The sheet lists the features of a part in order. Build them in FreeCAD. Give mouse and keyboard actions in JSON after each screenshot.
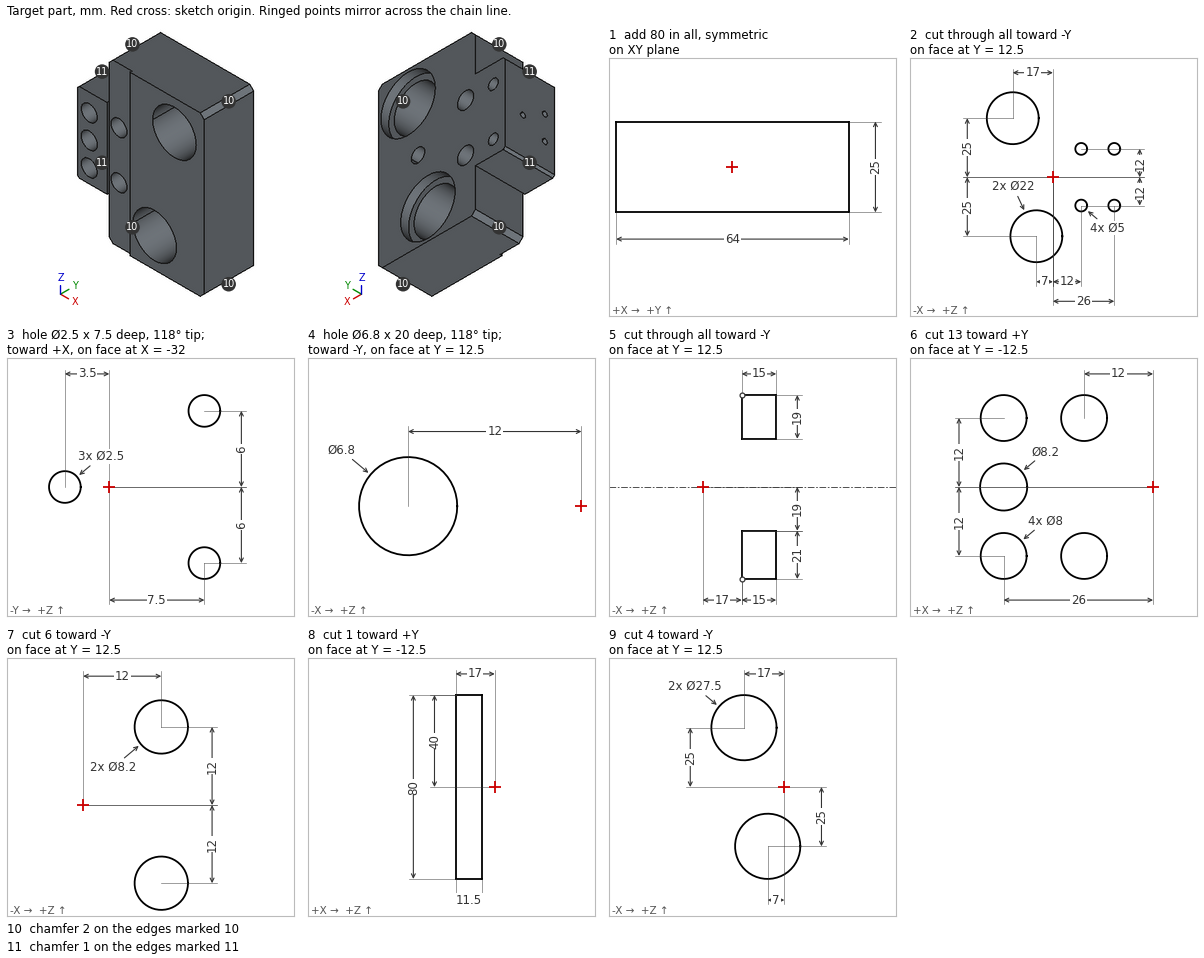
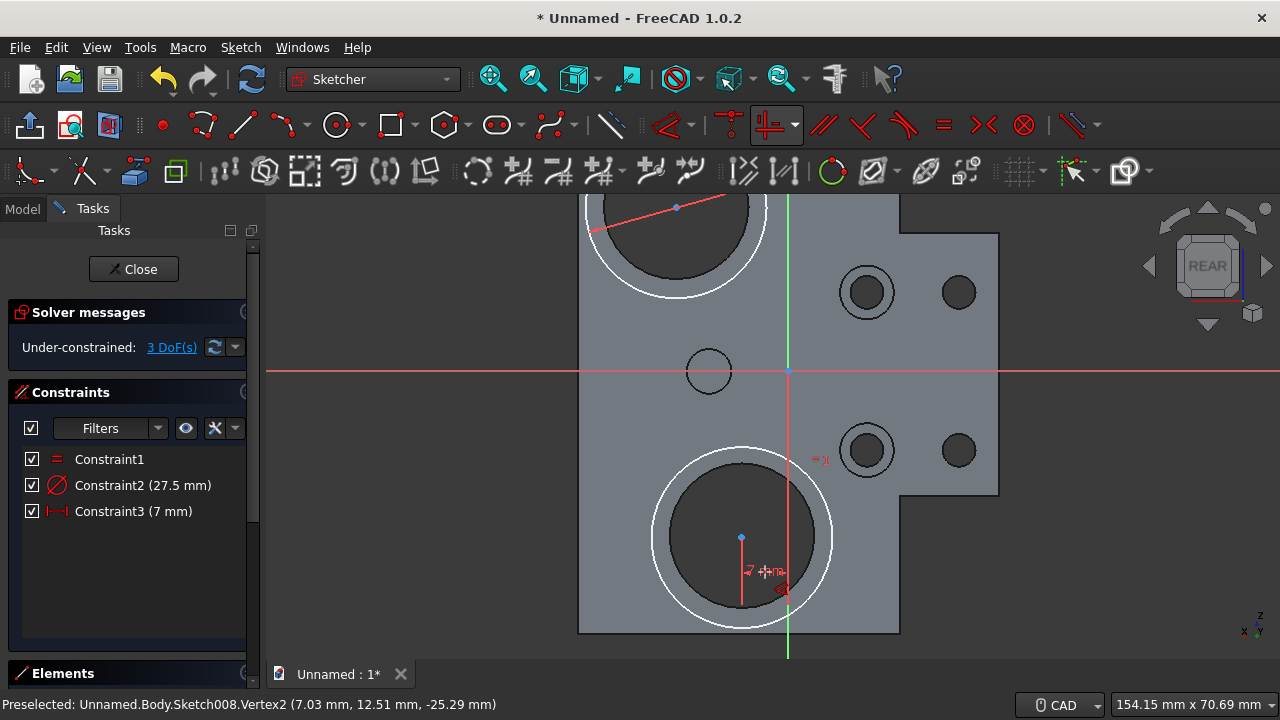
{"action": "scroll", "coordinate": [699, 494], "scroll_direction": "down", "scroll_amount": 3}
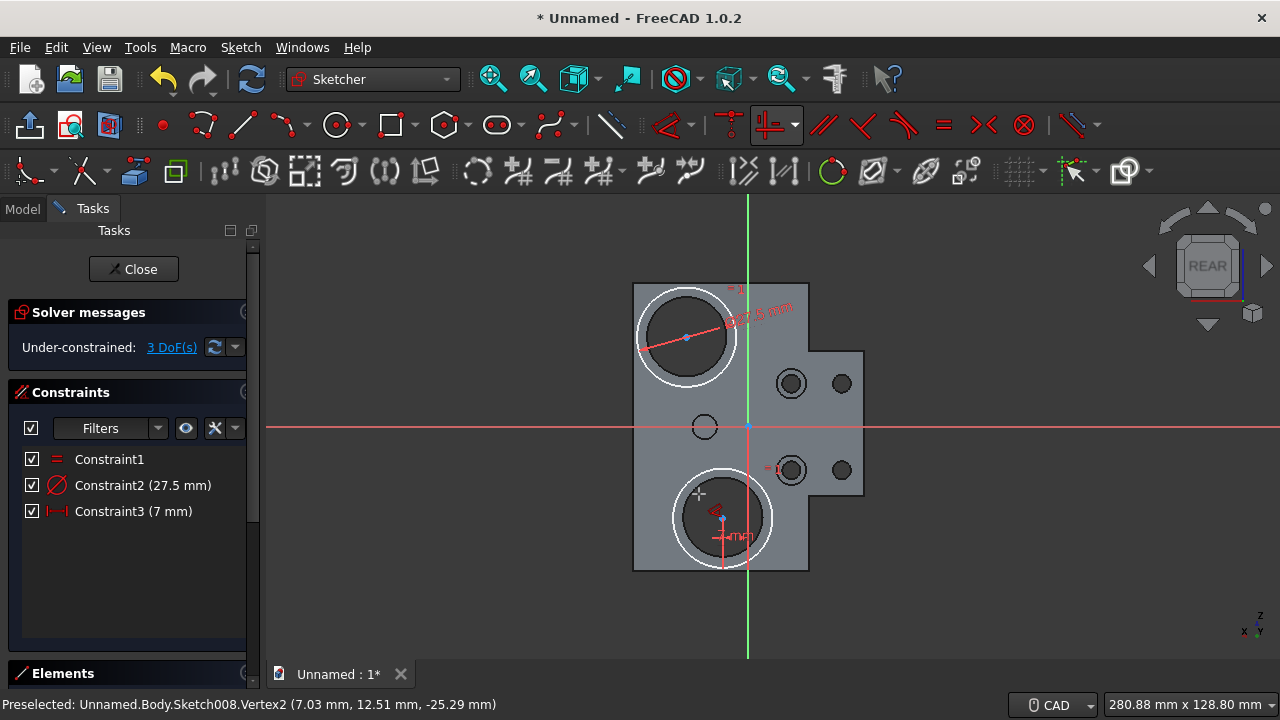
{"action": "left_click", "coordinate": [687, 337]}
{"action": "left_click", "coordinate": [696, 461]}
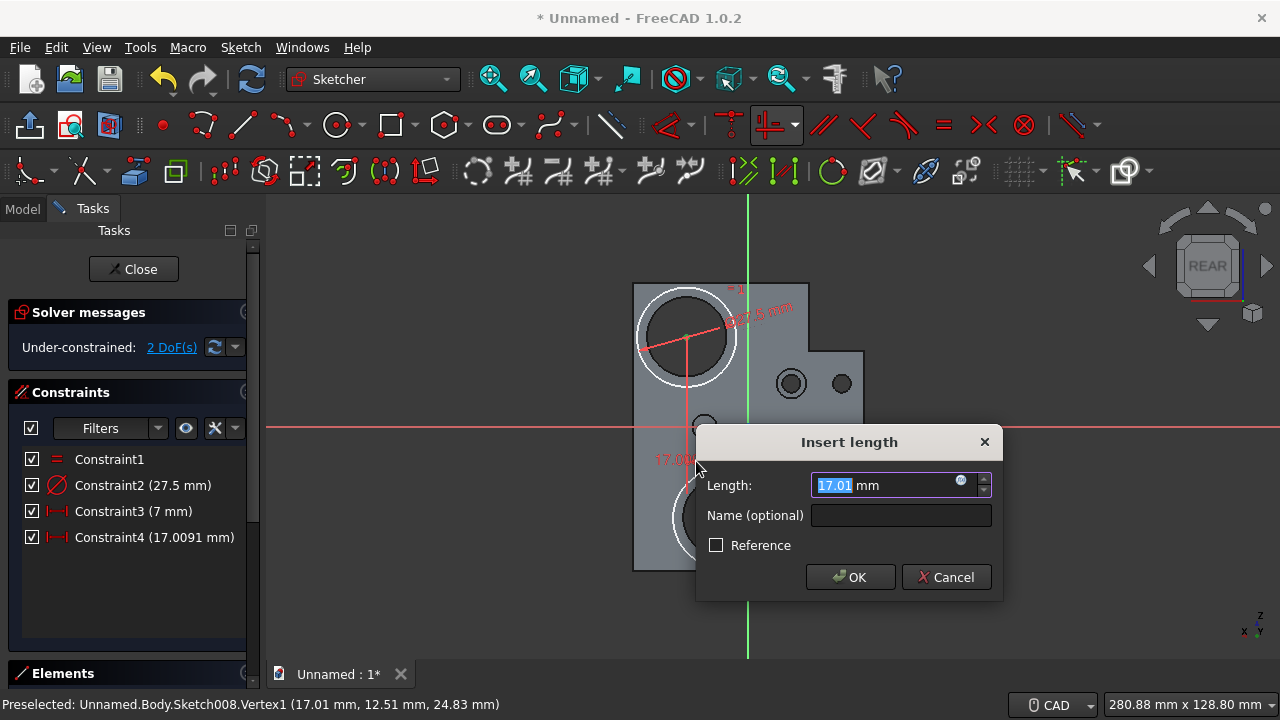
{"action": "type", "text": "17"}
{"action": "key", "text": "Return"}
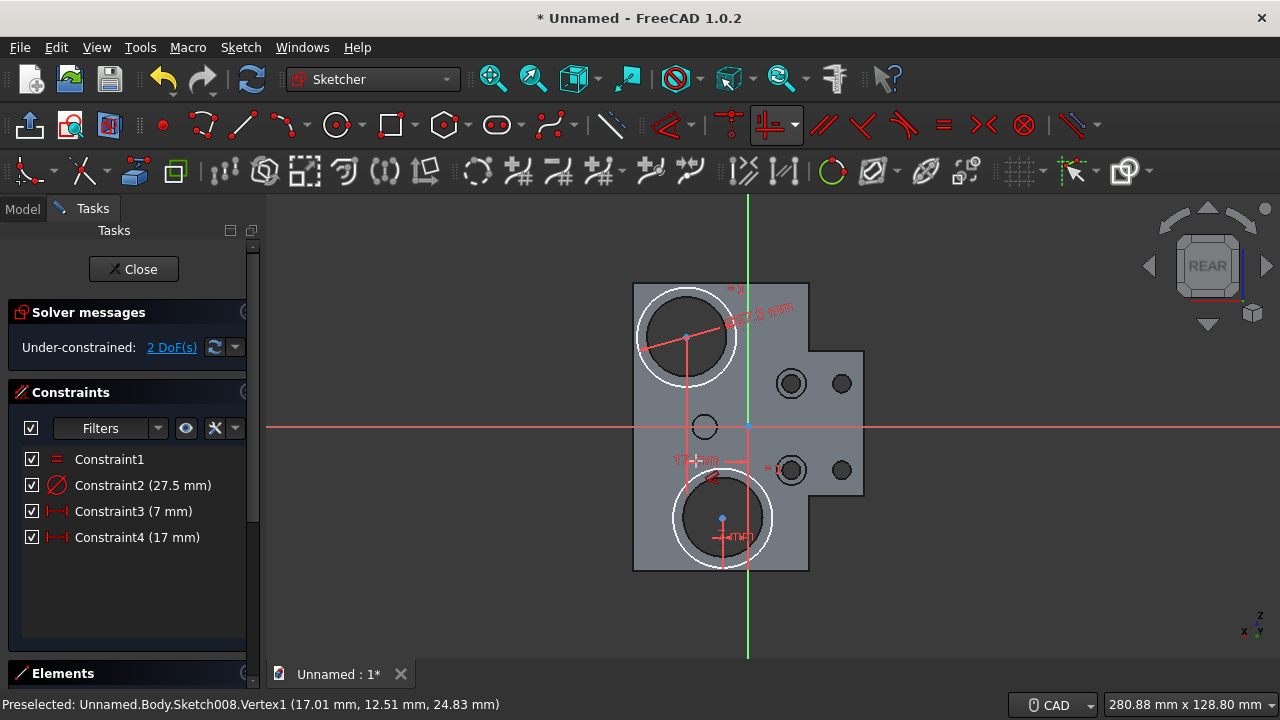
{"action": "left_click", "coordinate": [687, 337]}
{"action": "left_click", "coordinate": [782, 382]}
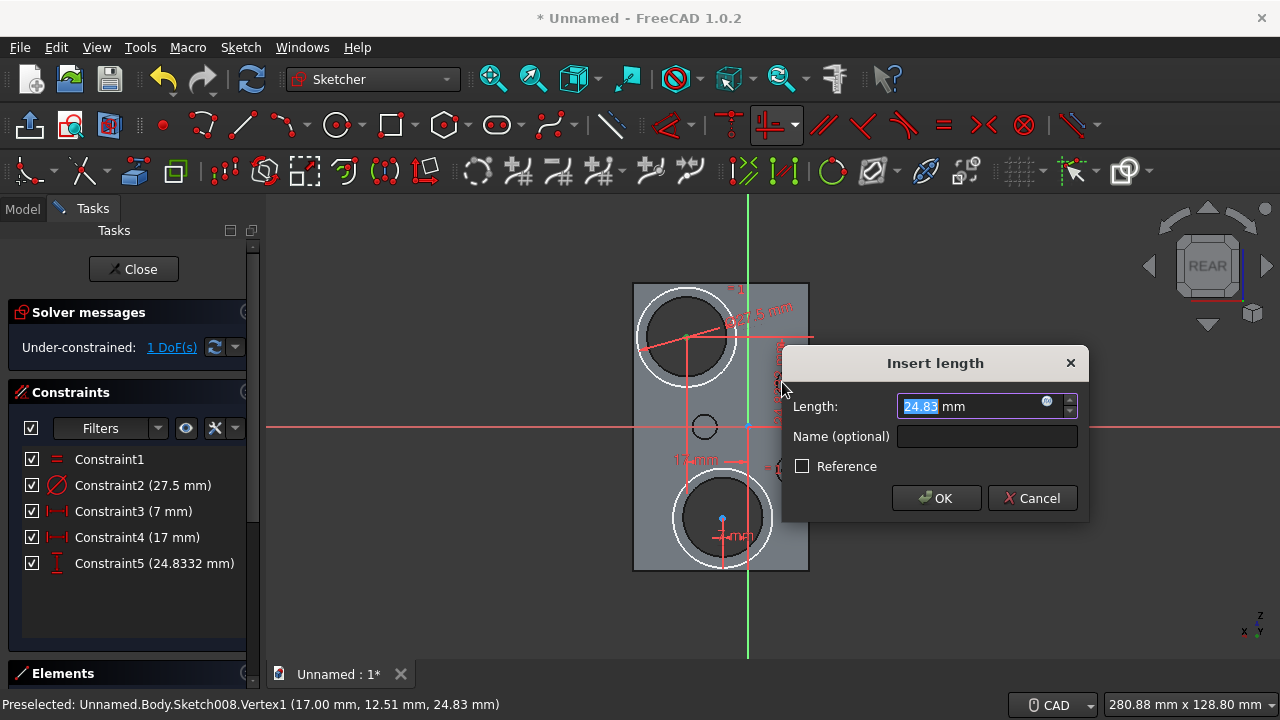
{"action": "type", "text": "25"}
{"action": "key", "text": "Return"}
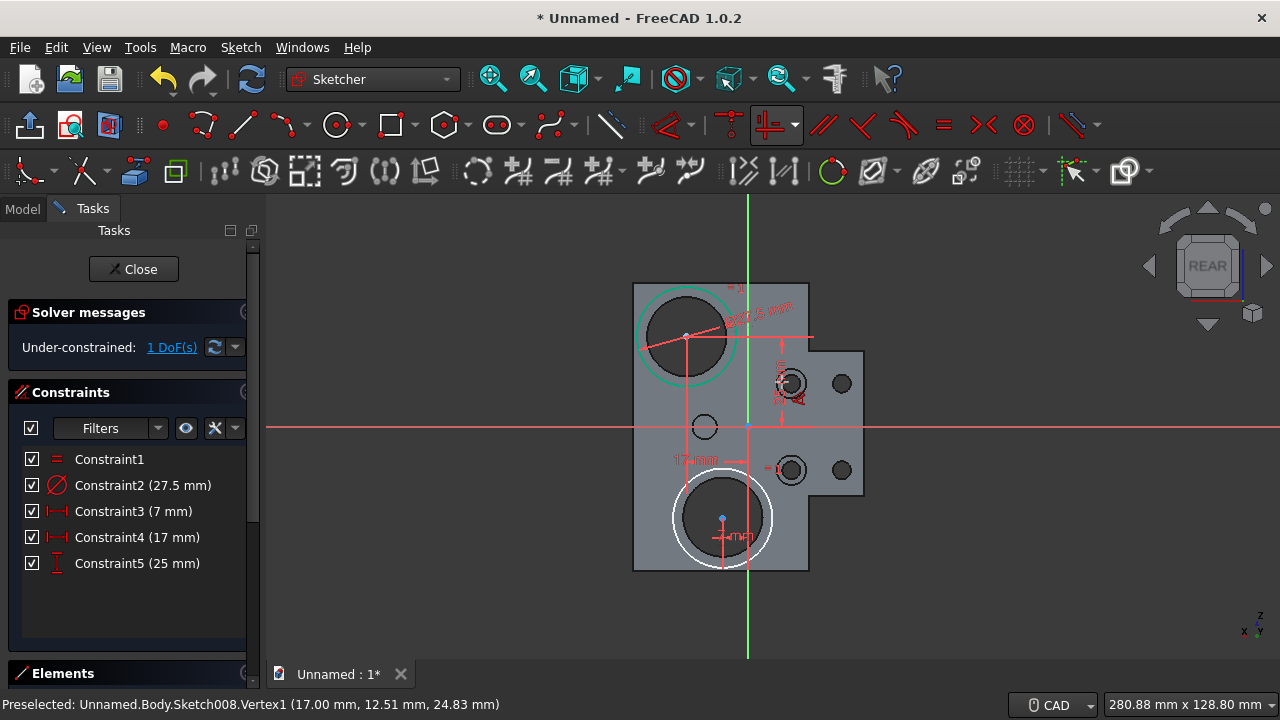
{"action": "left_click", "coordinate": [723, 518]}
{"action": "left_click", "coordinate": [782, 473]}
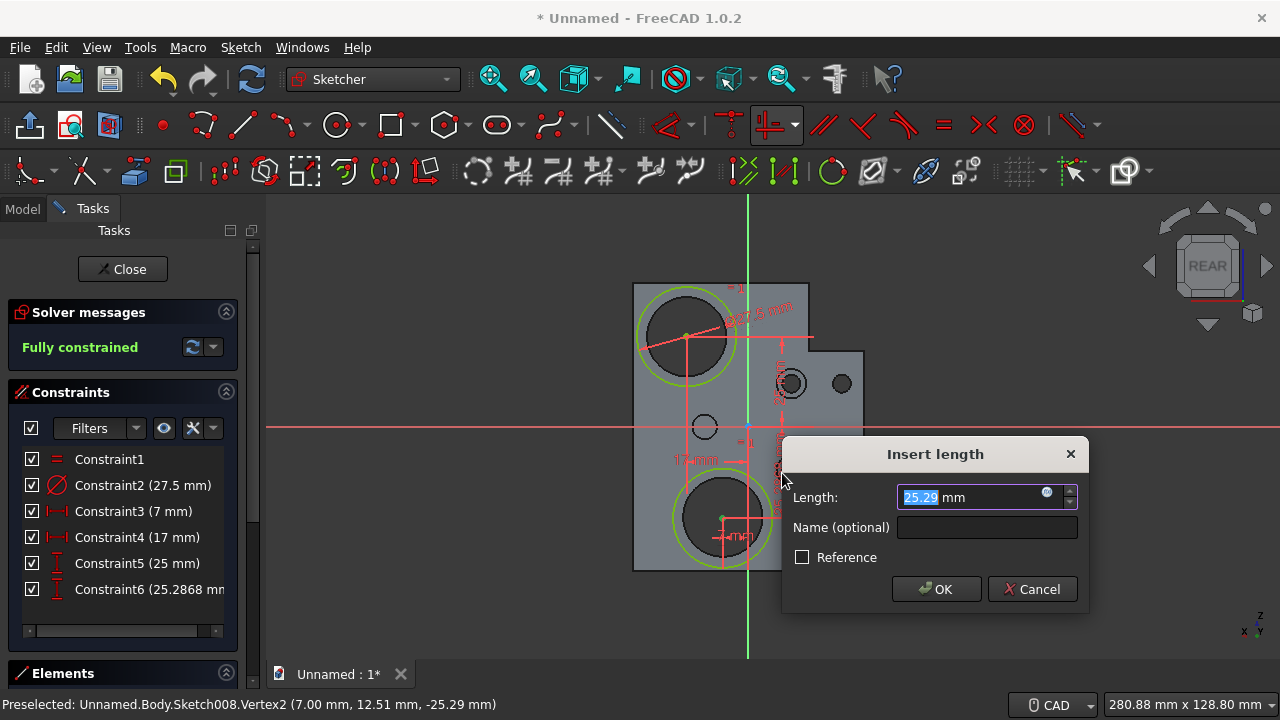
{"action": "type", "text": "25"}
{"action": "key", "text": "Return"}
{"action": "key", "text": "Escape"}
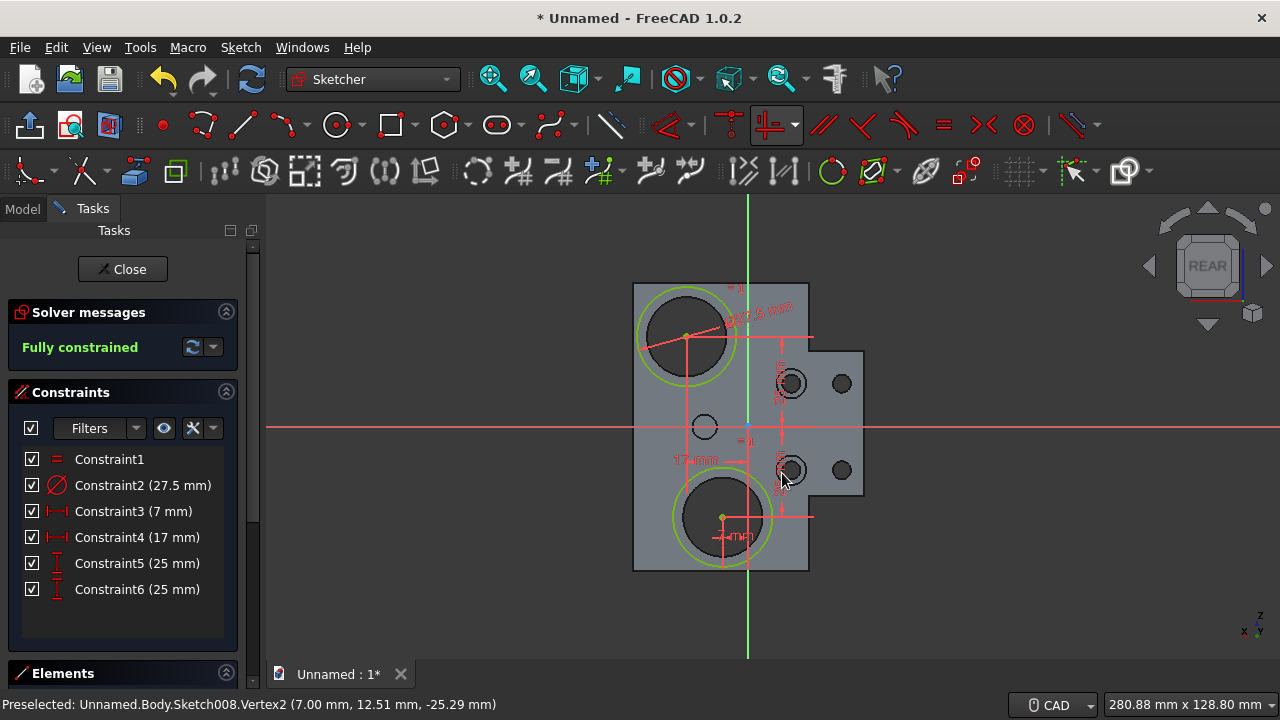
{"action": "left_click", "coordinate": [123, 269]}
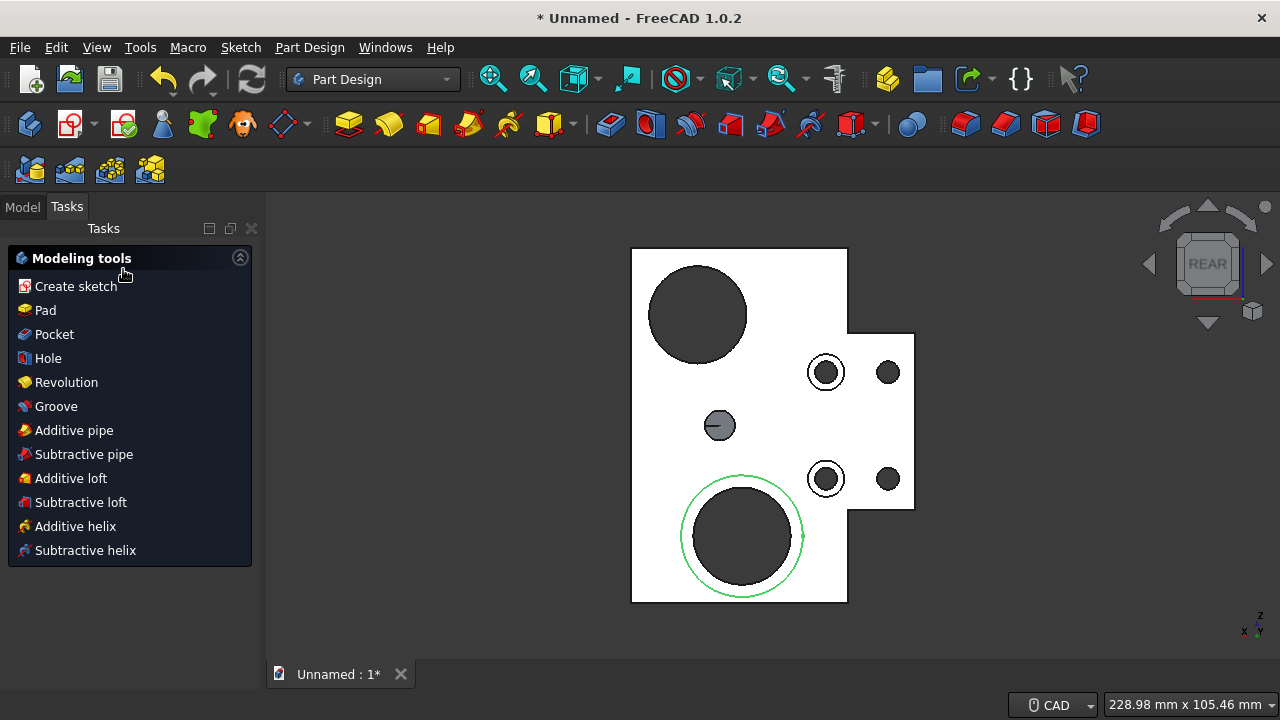
{"action": "left_click", "coordinate": [612, 124]}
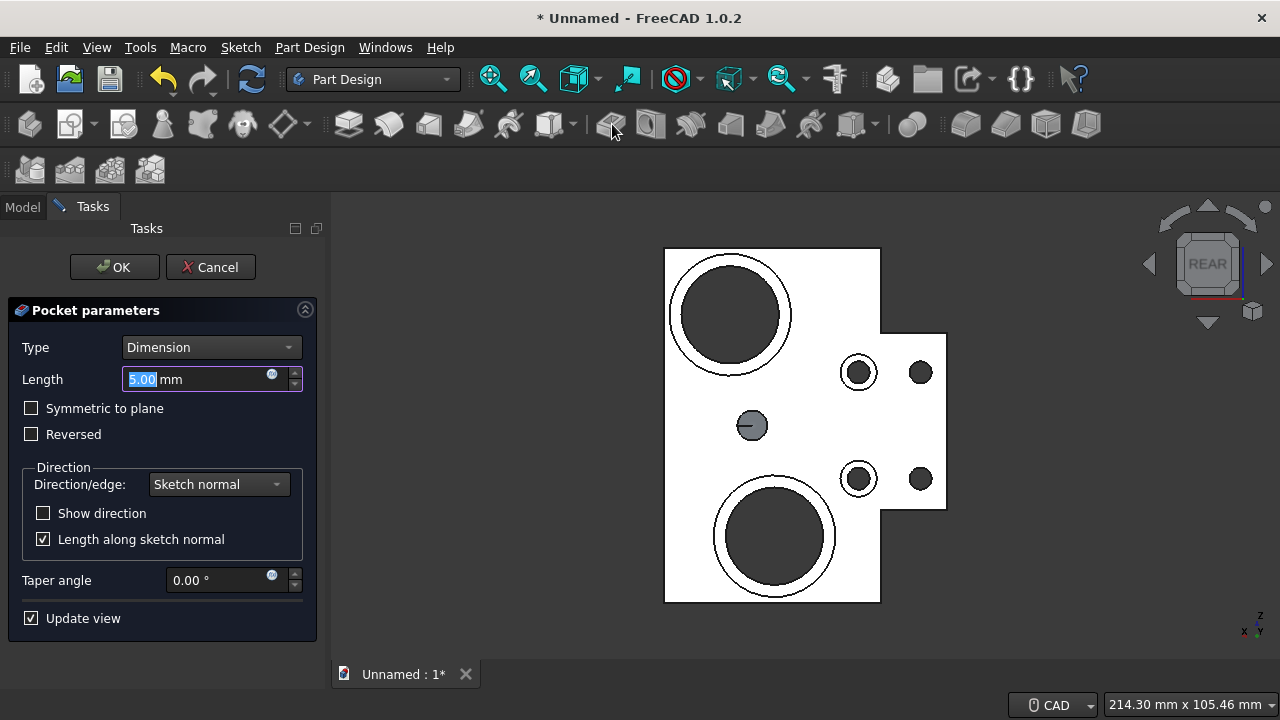
{"action": "type", "text": "4"}
{"action": "key", "text": "Tab"}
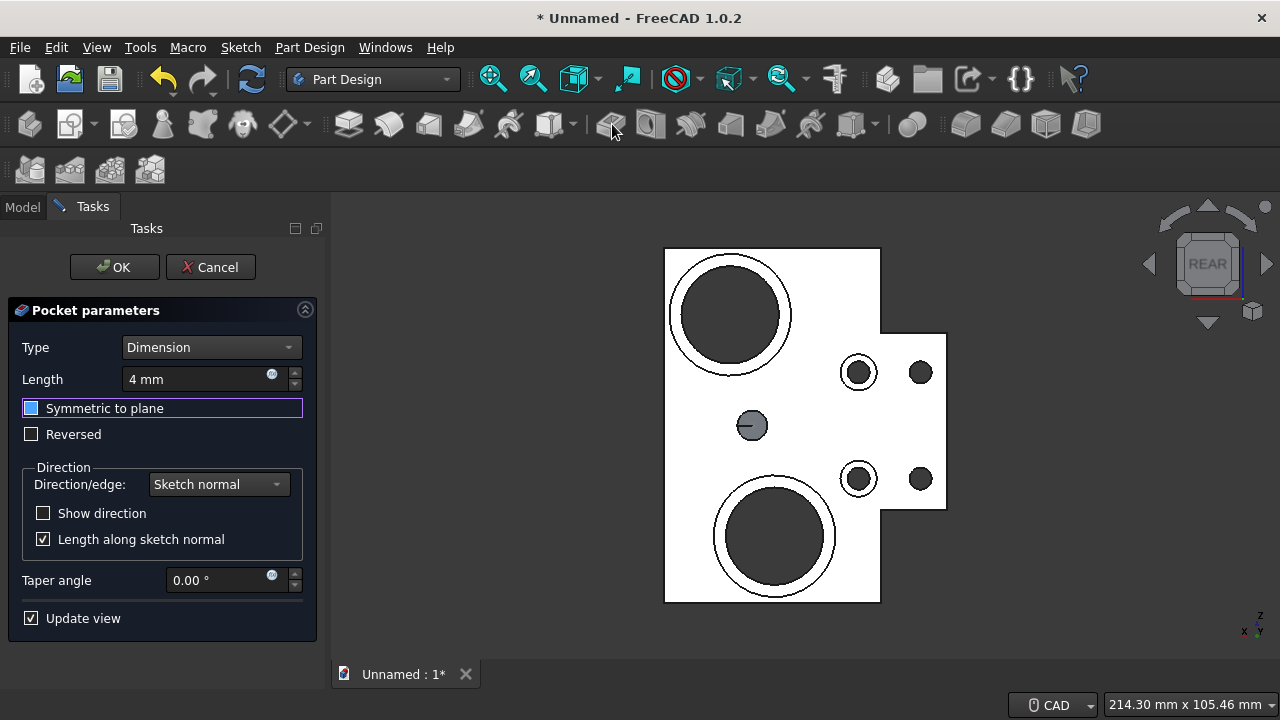
{"action": "left_click", "coordinate": [115, 267]}